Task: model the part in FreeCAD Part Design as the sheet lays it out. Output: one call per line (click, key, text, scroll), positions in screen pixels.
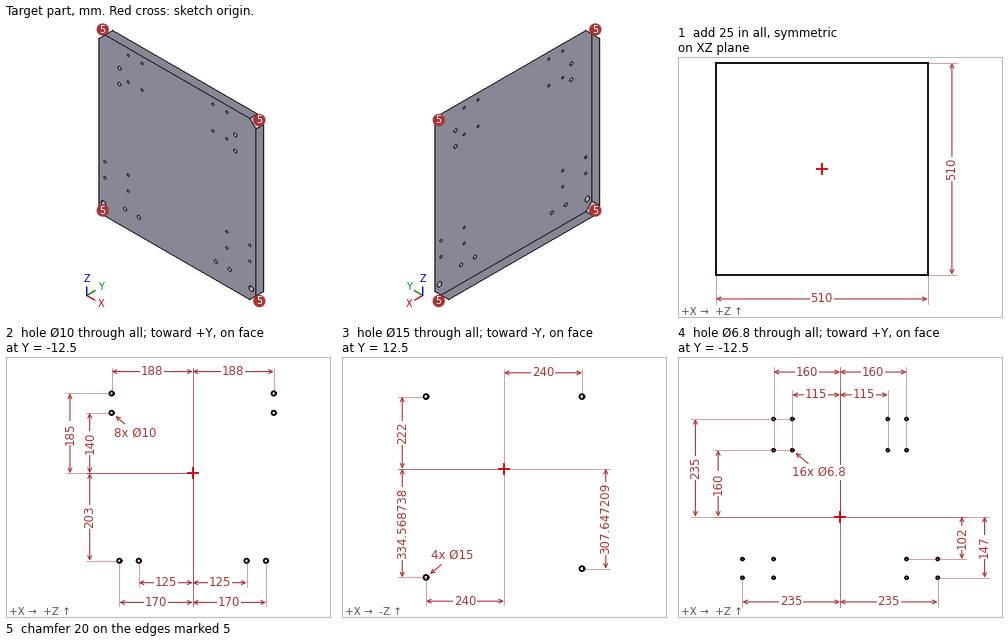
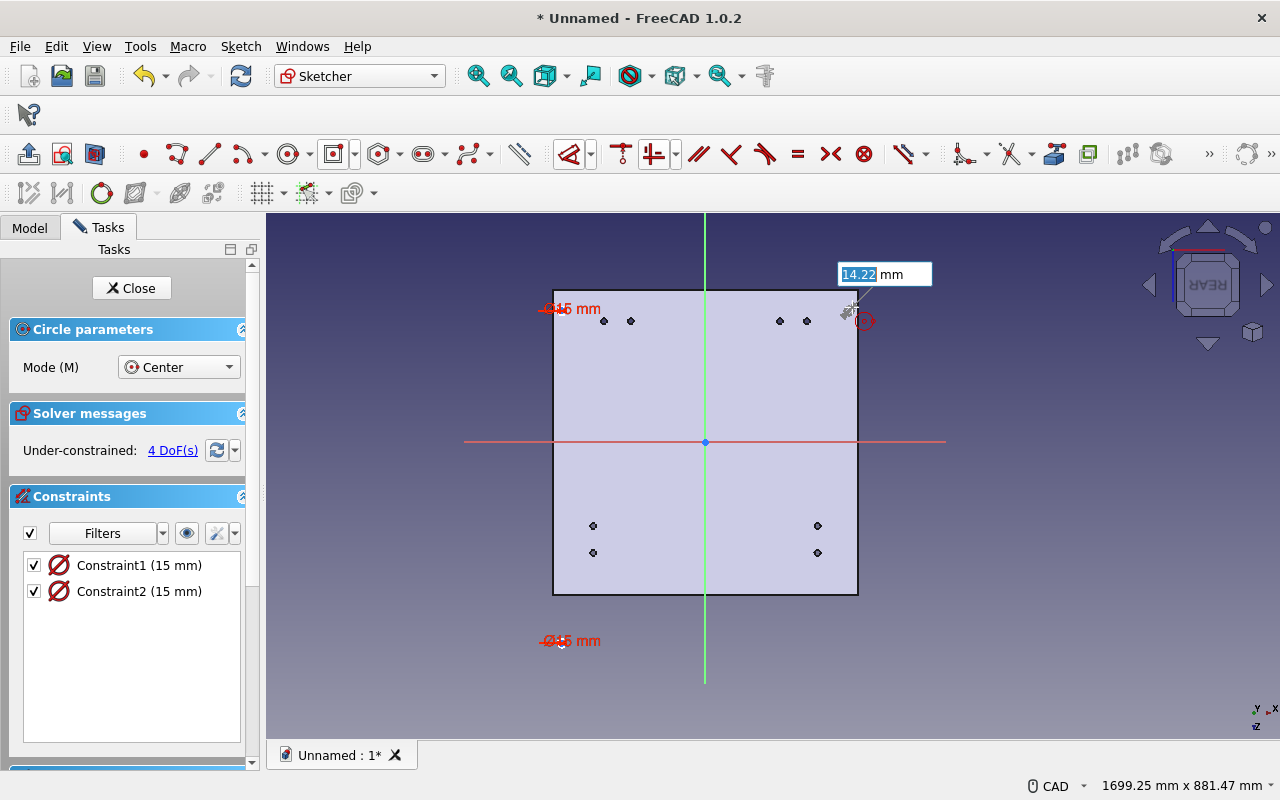
text(15)
key(Return)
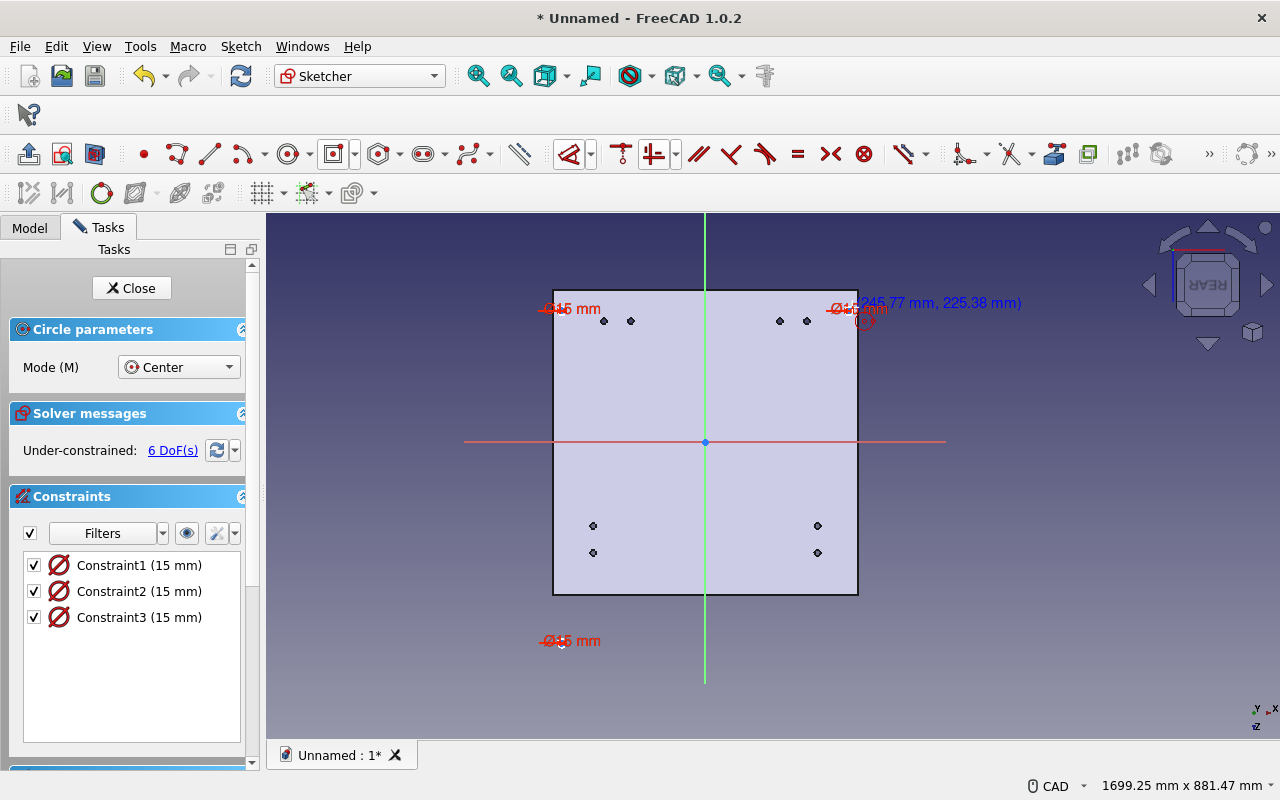
scroll(849, 626, up, 9)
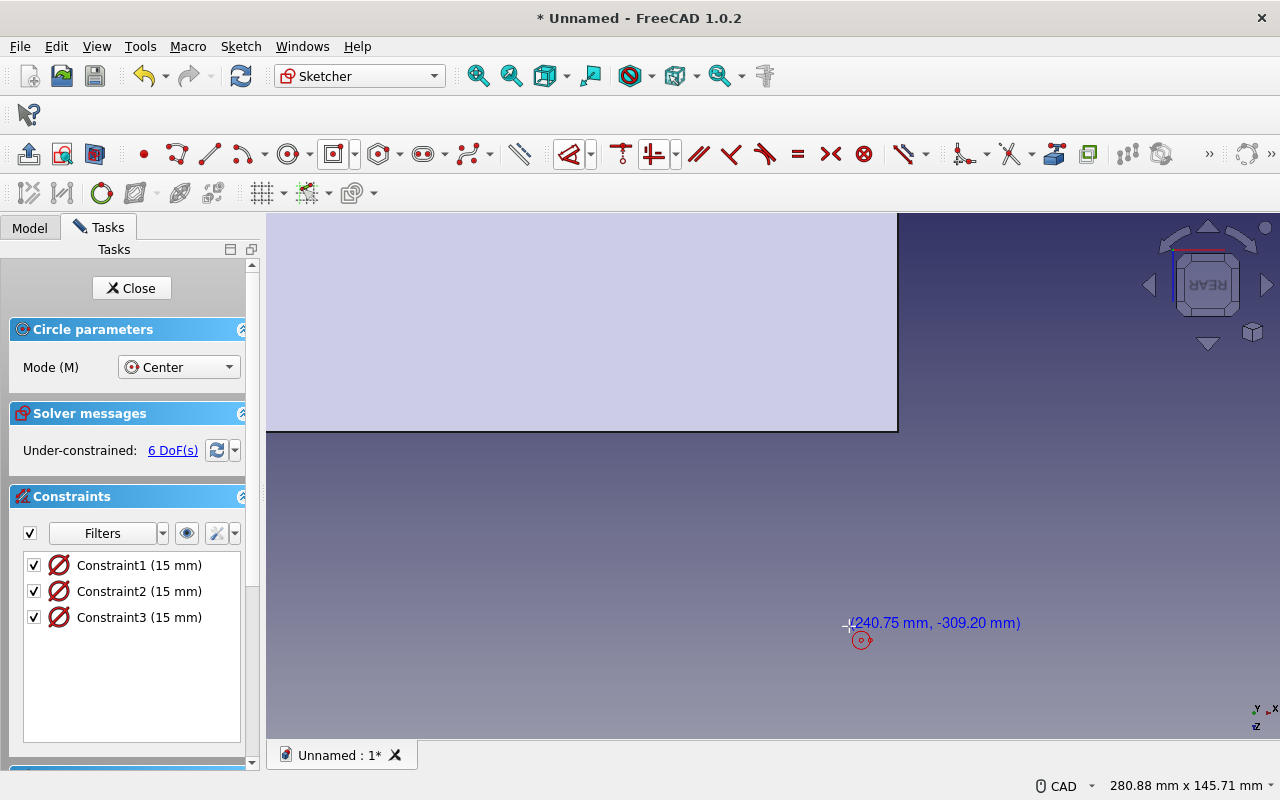
scroll(849, 627, down, 9)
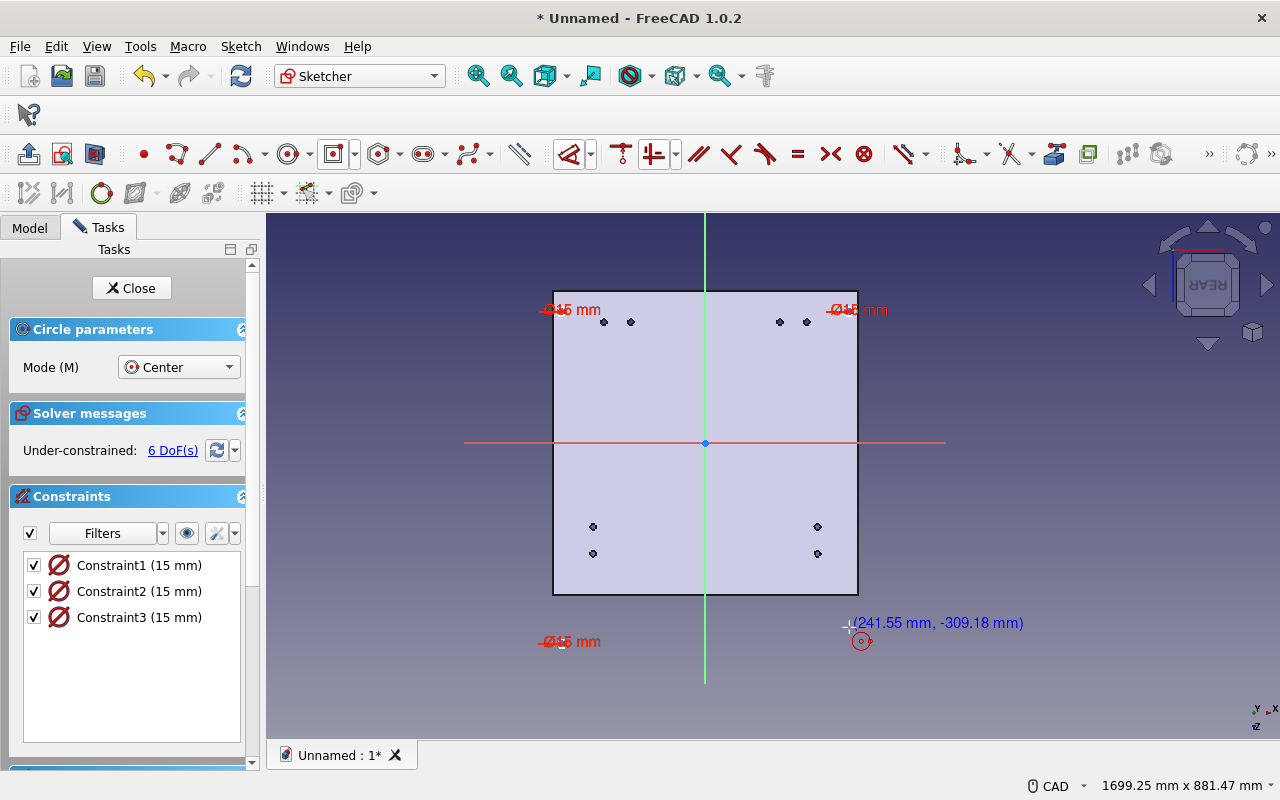
click(849, 627)
move(852, 624)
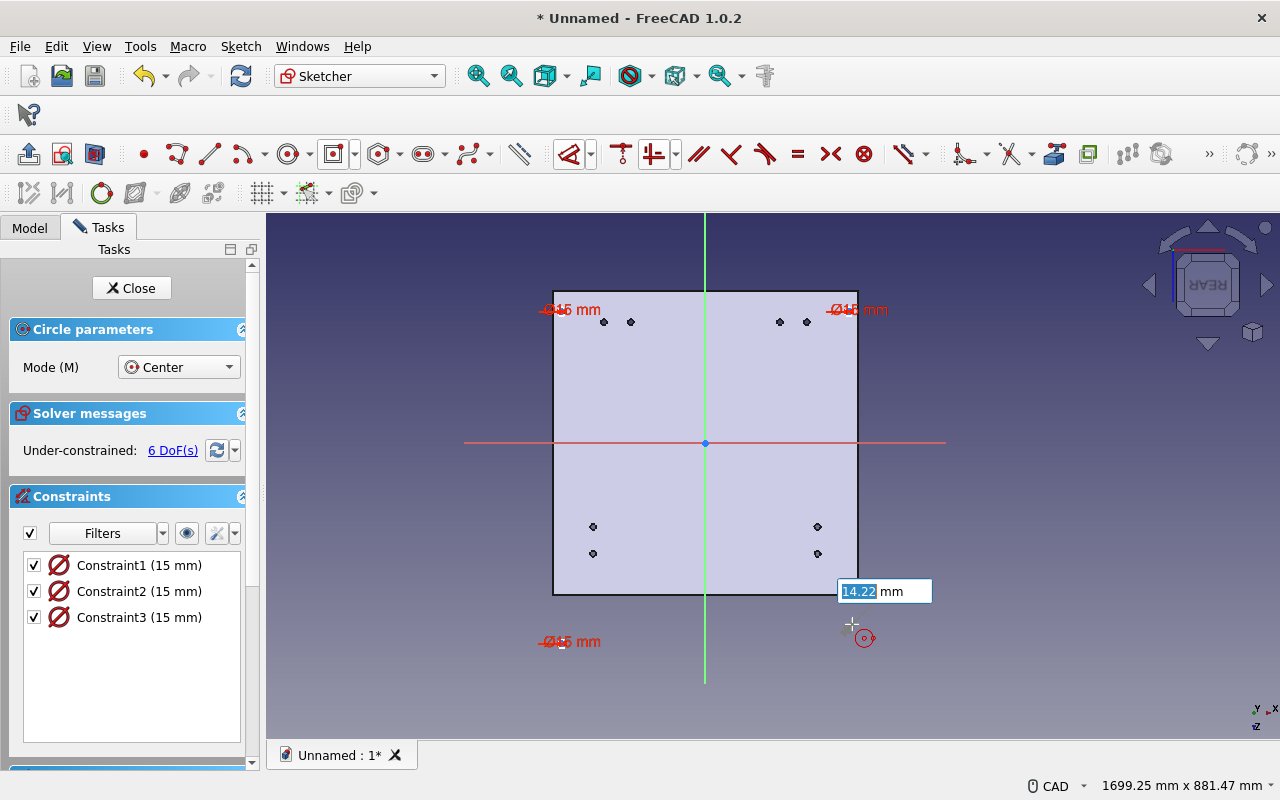
text(15)
key(Return)
key(Escape)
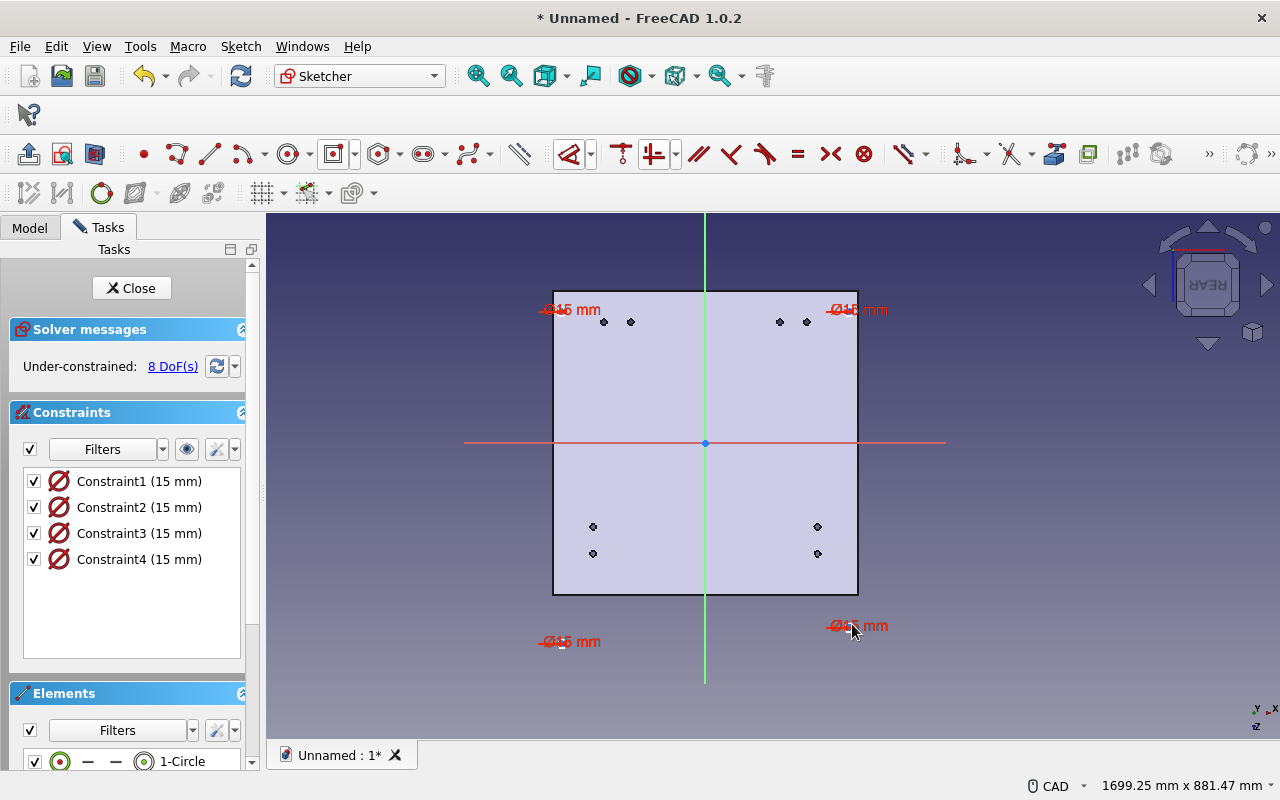
click(562, 644)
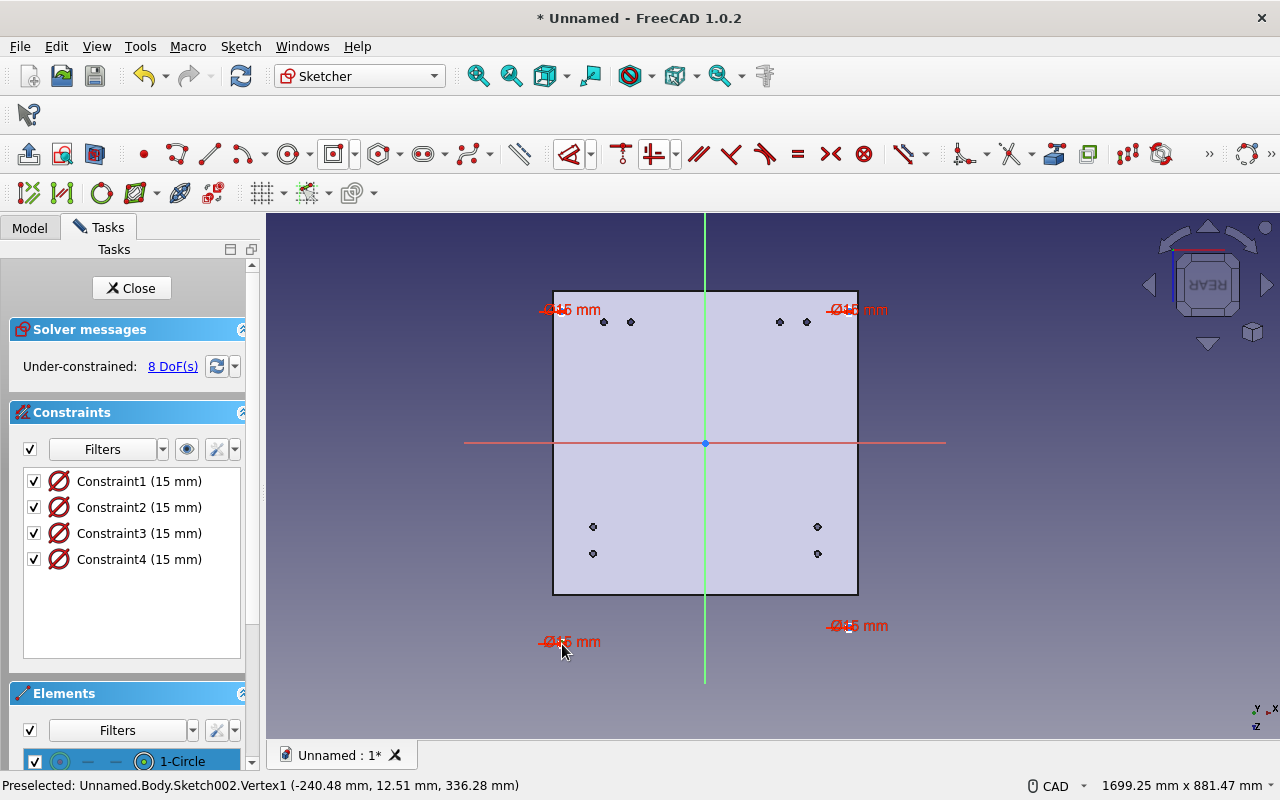
click(562, 312)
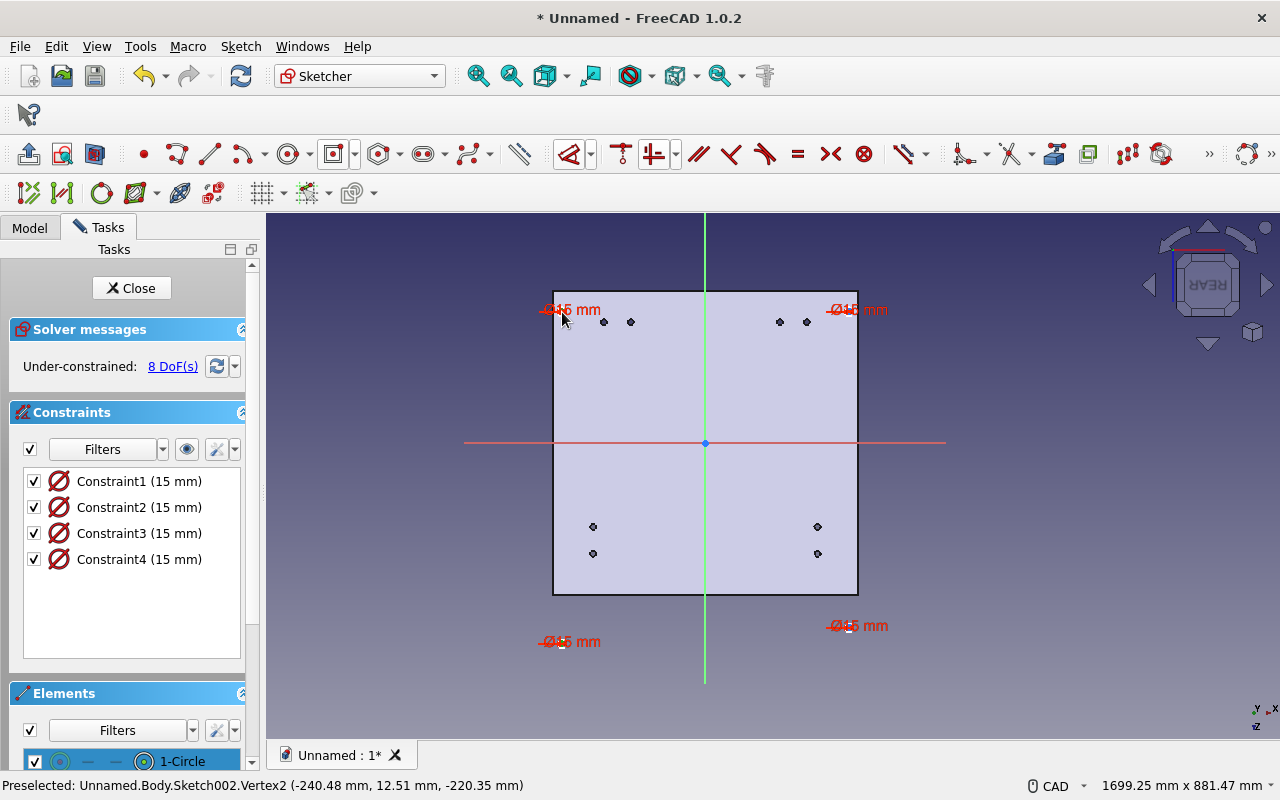
click(676, 154)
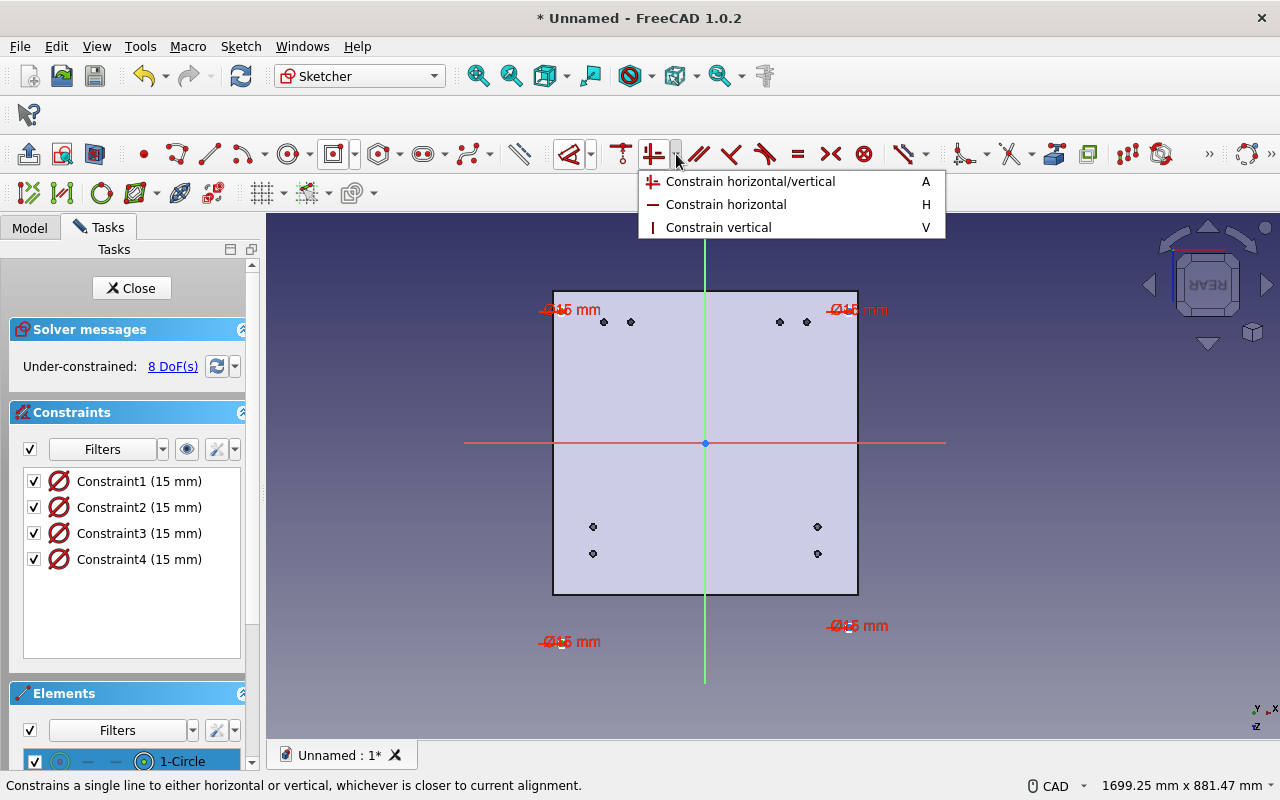
click(792, 228)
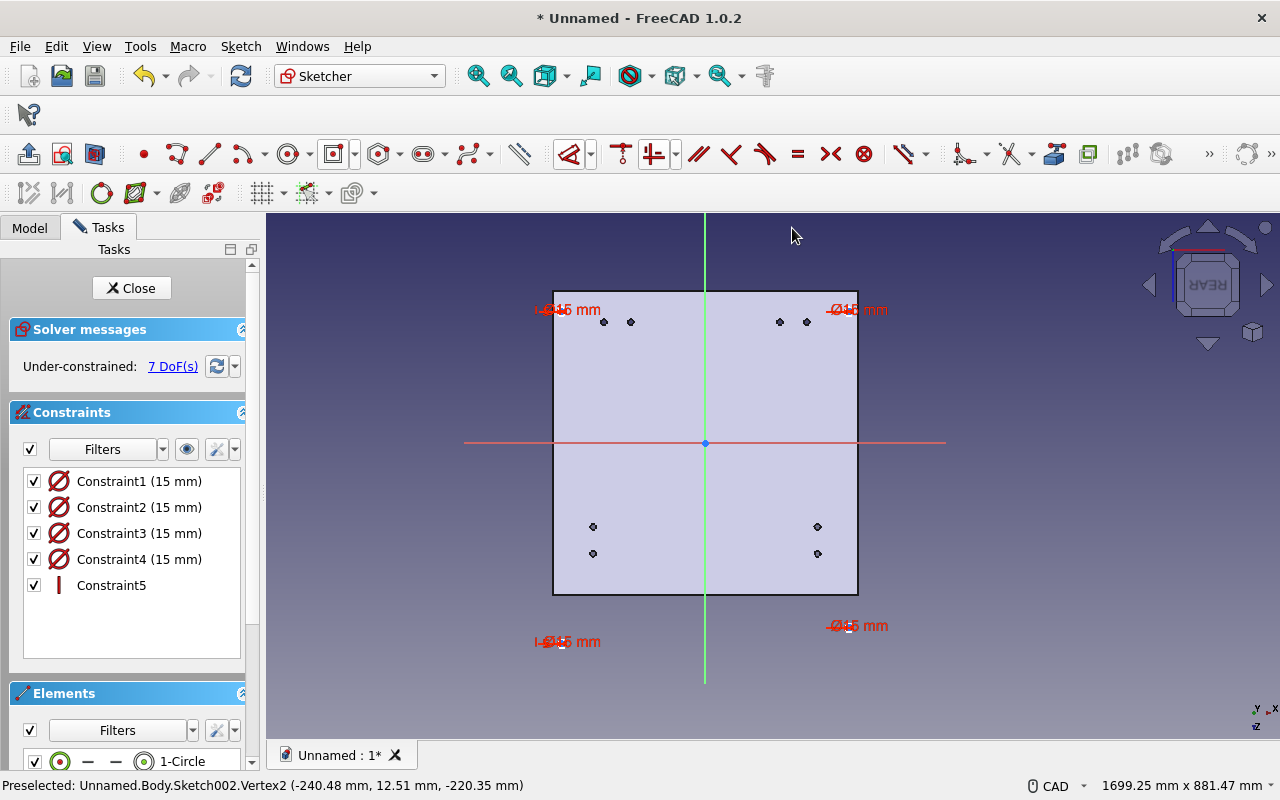
click(562, 312)